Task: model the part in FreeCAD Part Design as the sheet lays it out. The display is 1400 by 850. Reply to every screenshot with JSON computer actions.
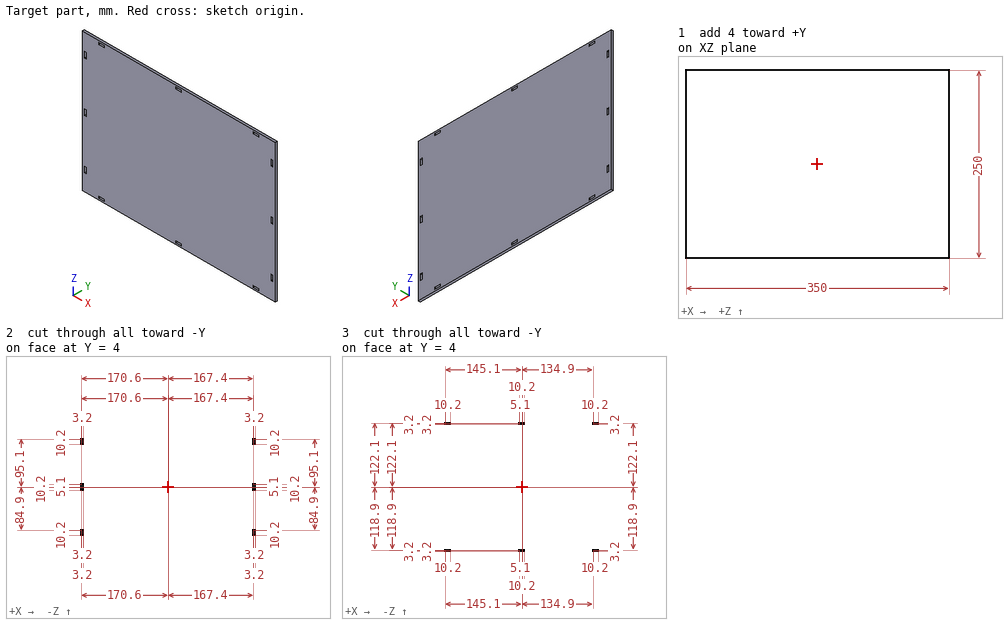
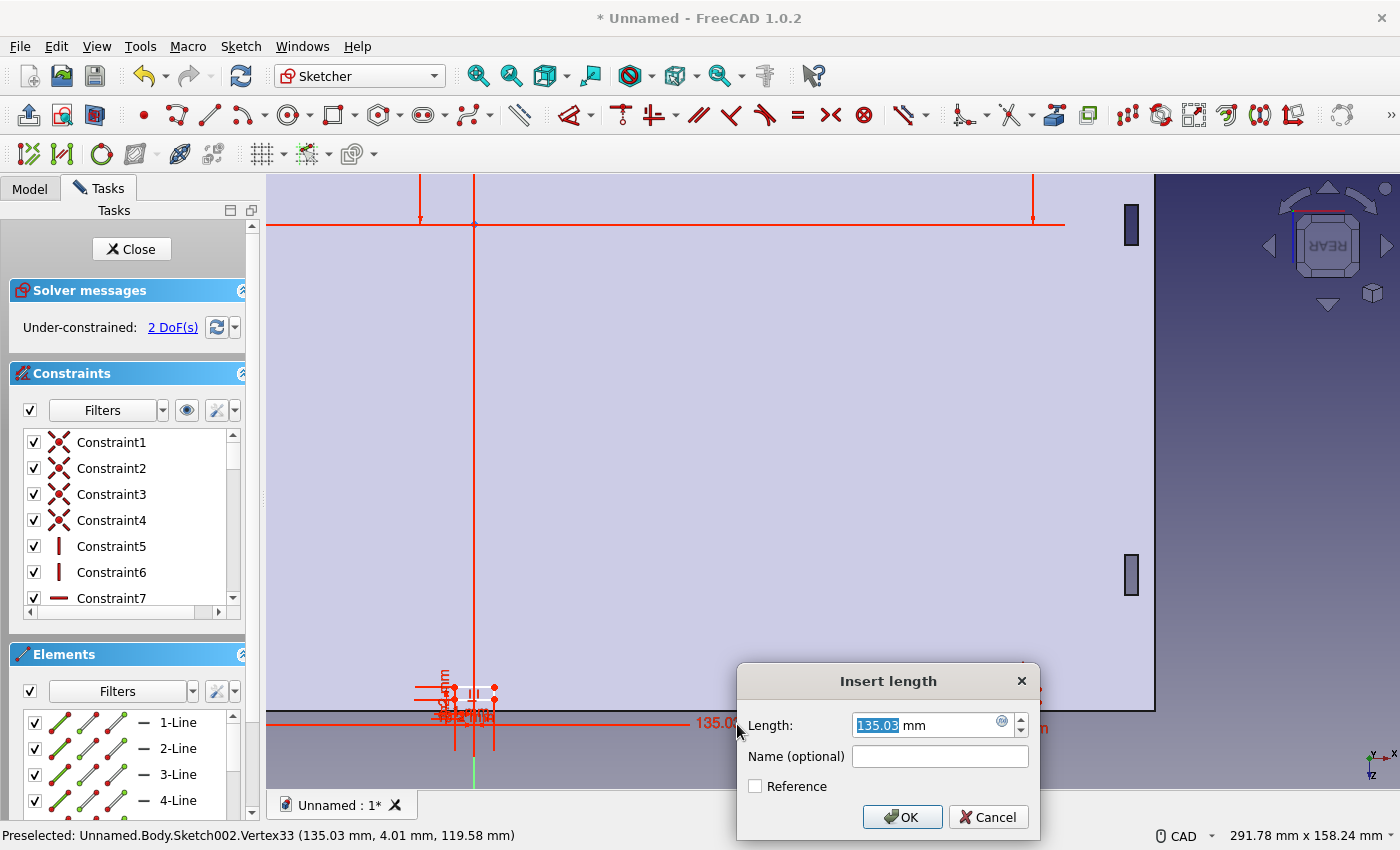
{"action": "type", "text": "134.9"}
{"action": "key", "text": "Return"}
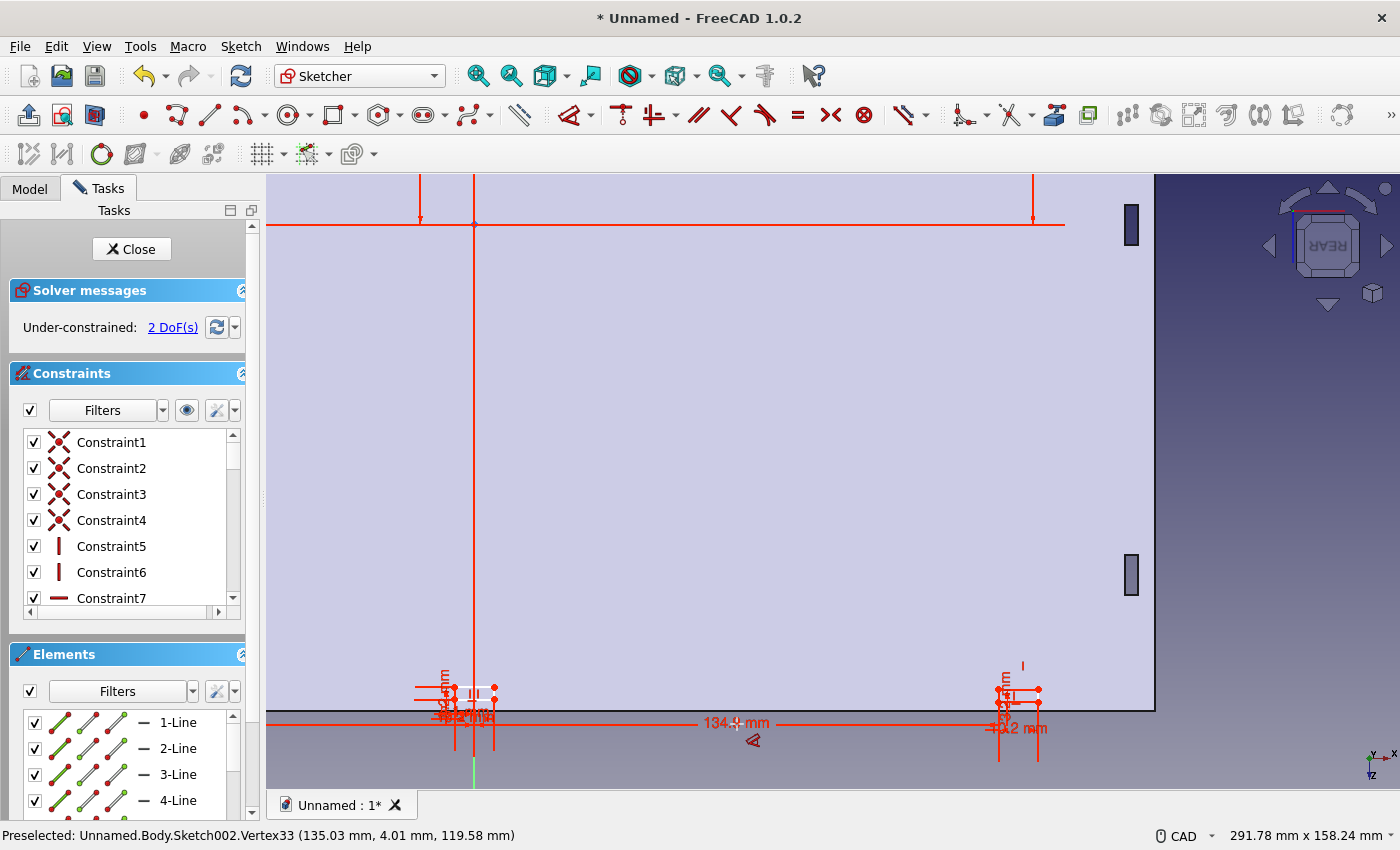
{"action": "left_click", "coordinate": [999, 690]}
{"action": "left_click", "coordinate": [1033, 457]}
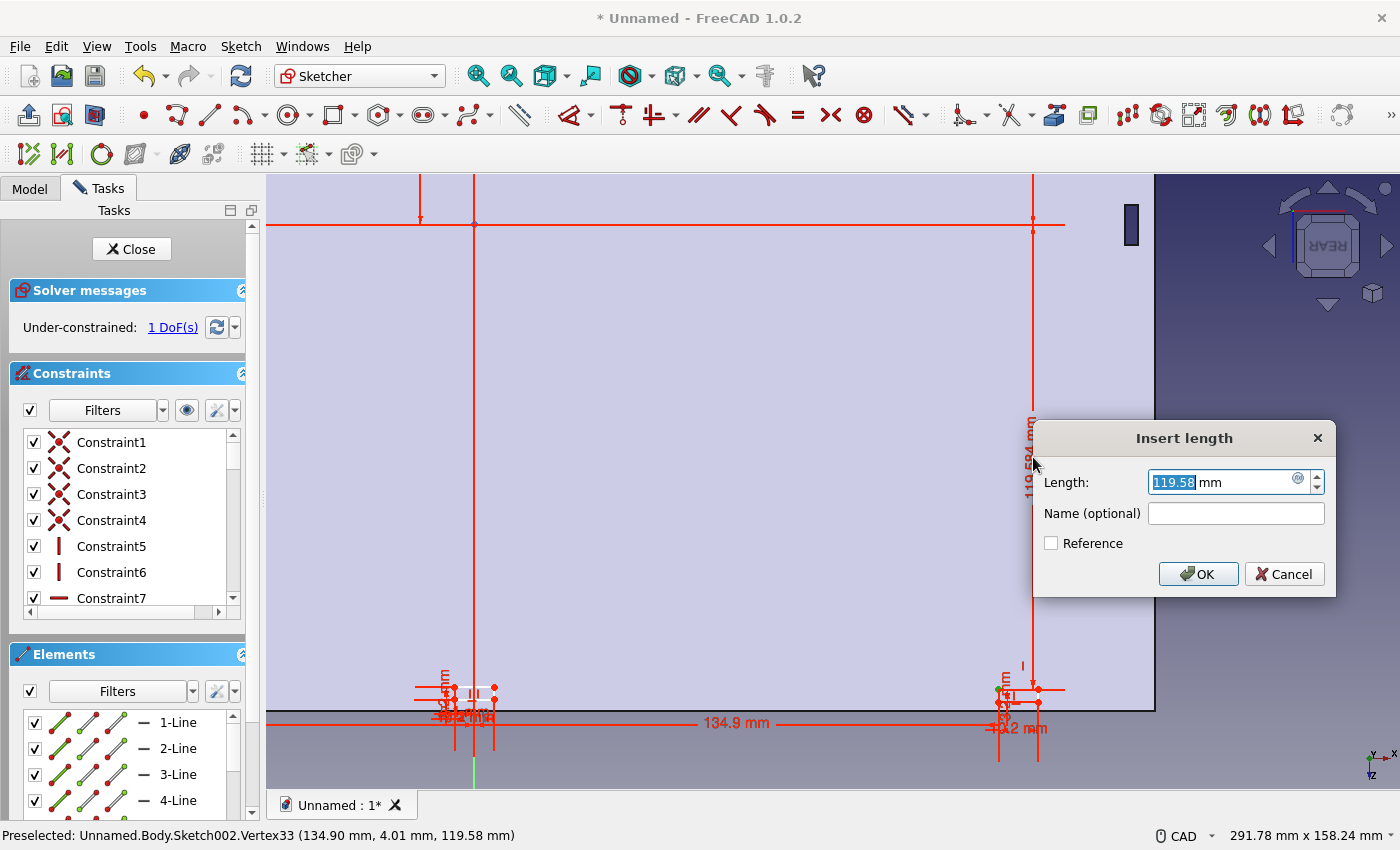
{"action": "type", "text": "118.9"}
{"action": "key", "text": "Return"}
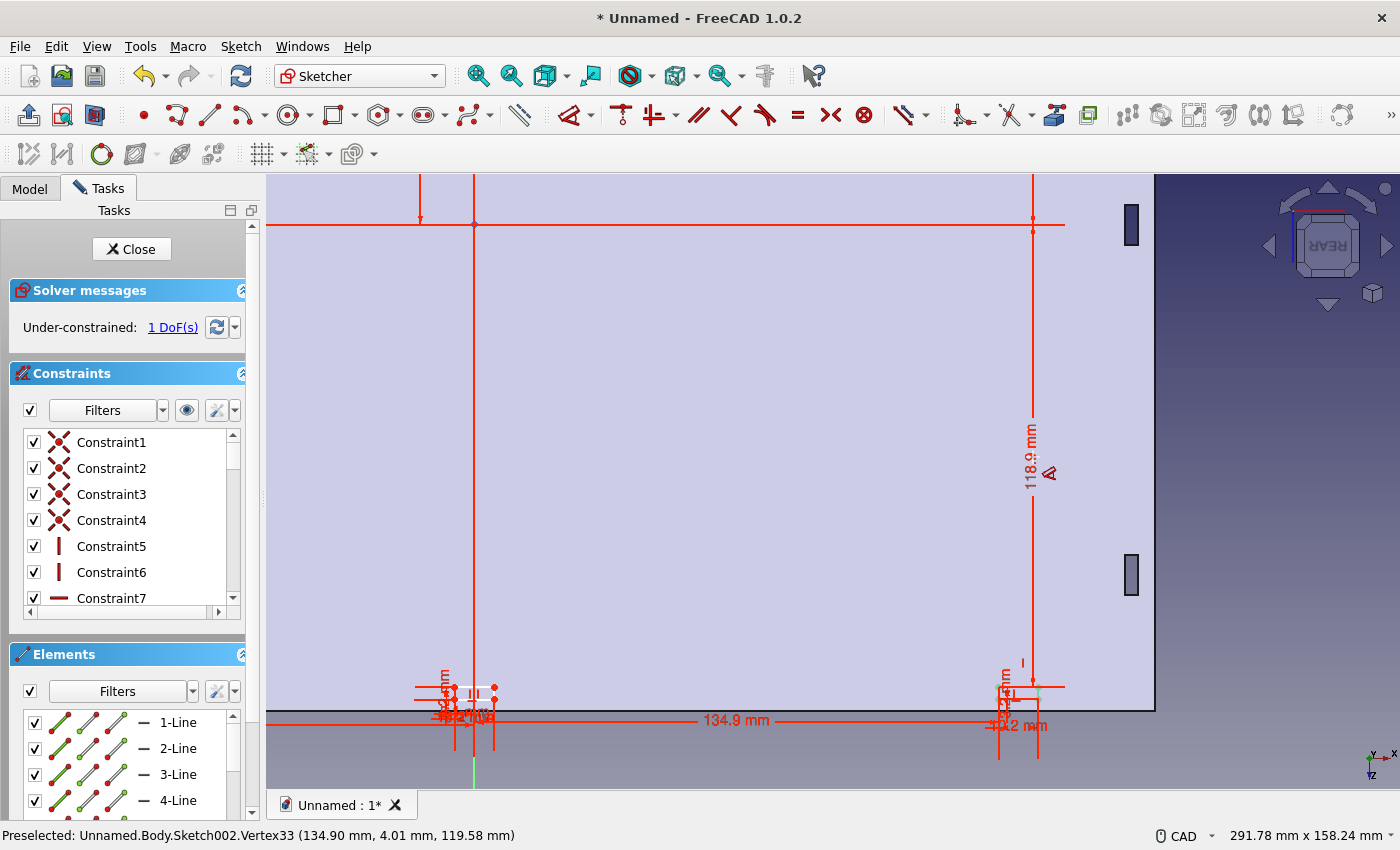
{"action": "left_click", "coordinate": [455, 687]}
{"action": "left_click", "coordinate": [421, 456]}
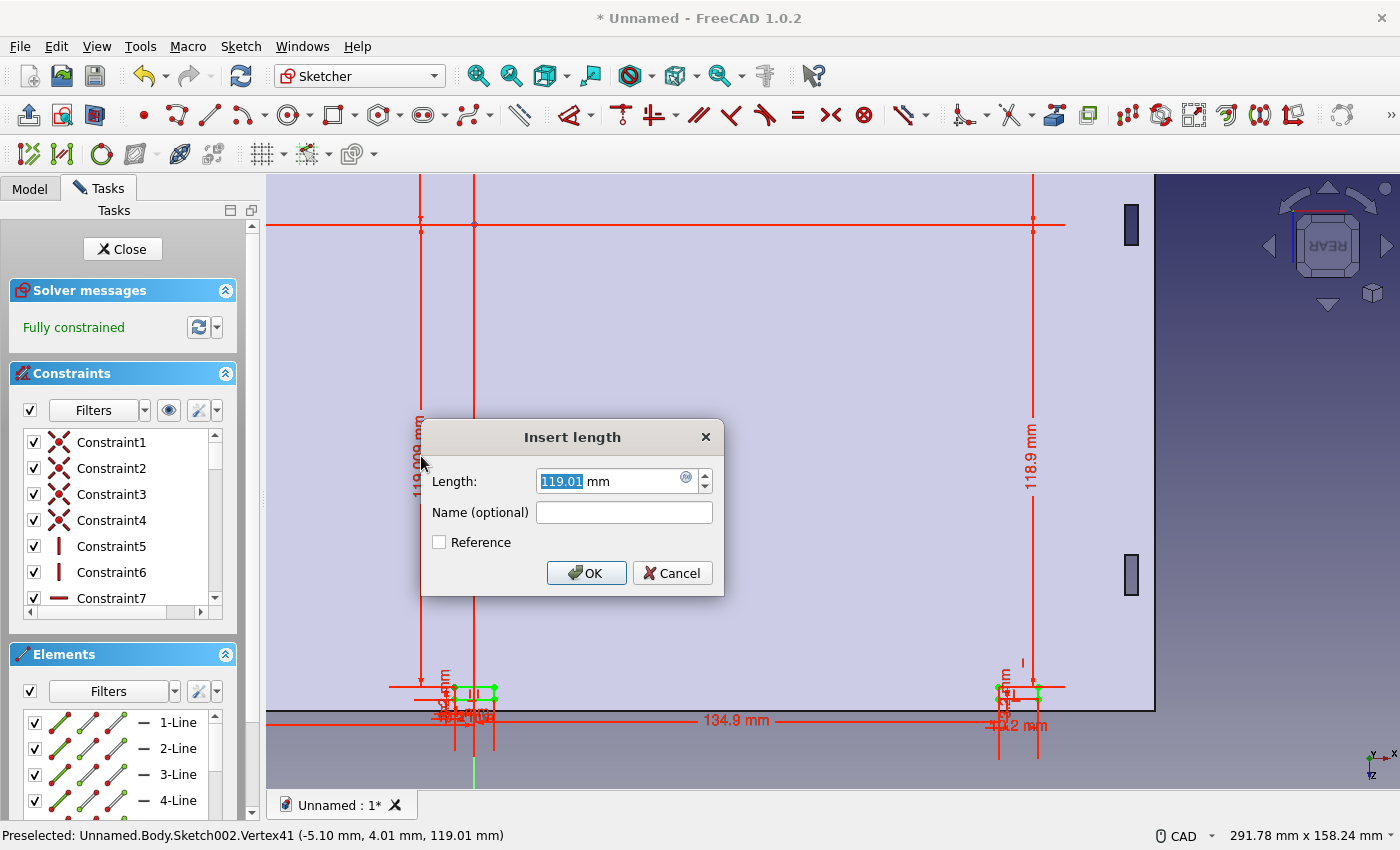
{"action": "type", "text": "118.9"}
{"action": "key", "text": "Return"}
{"action": "key", "text": "Escape"}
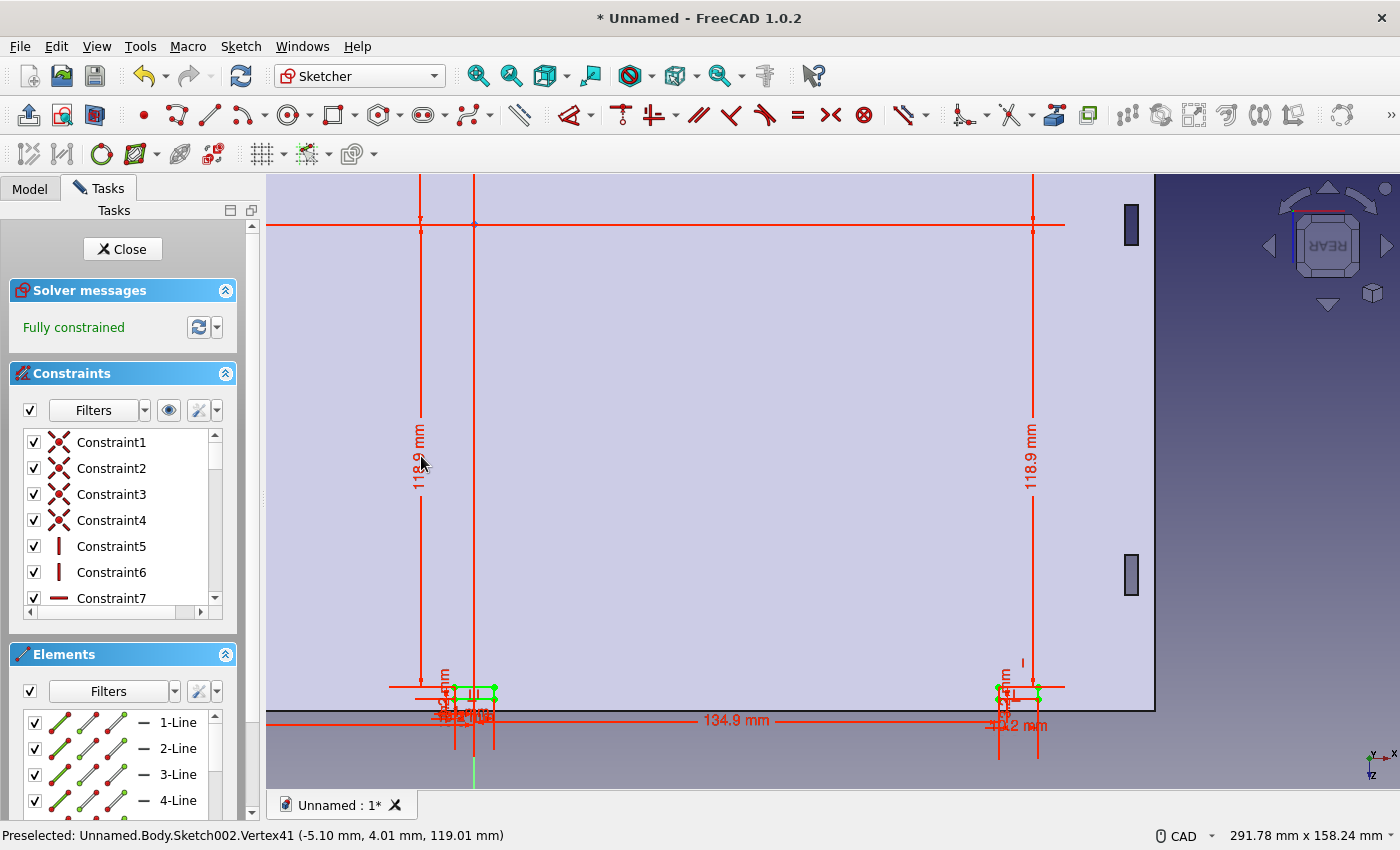
{"action": "left_click", "coordinate": [123, 249]}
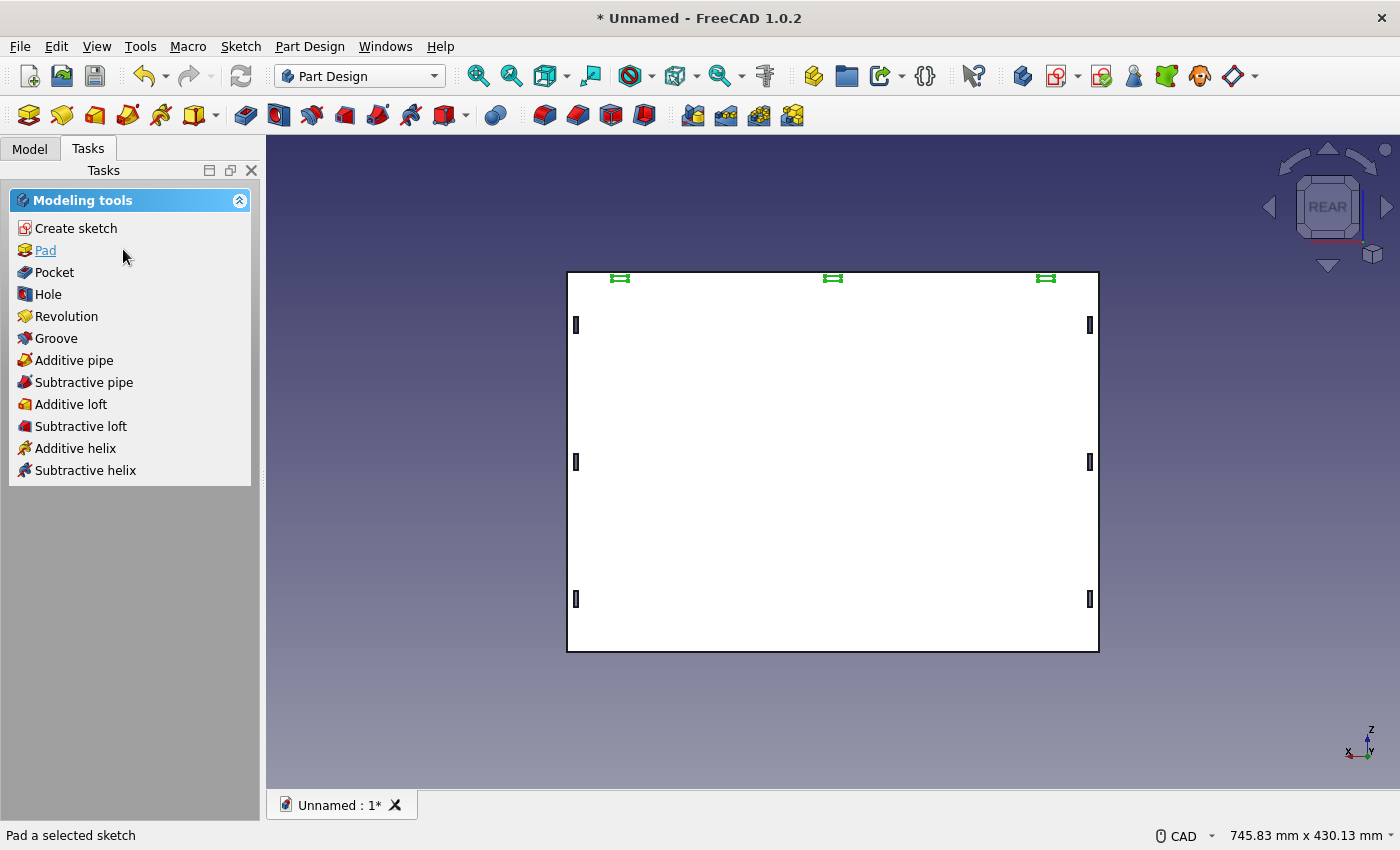
{"action": "left_click", "coordinate": [246, 116]}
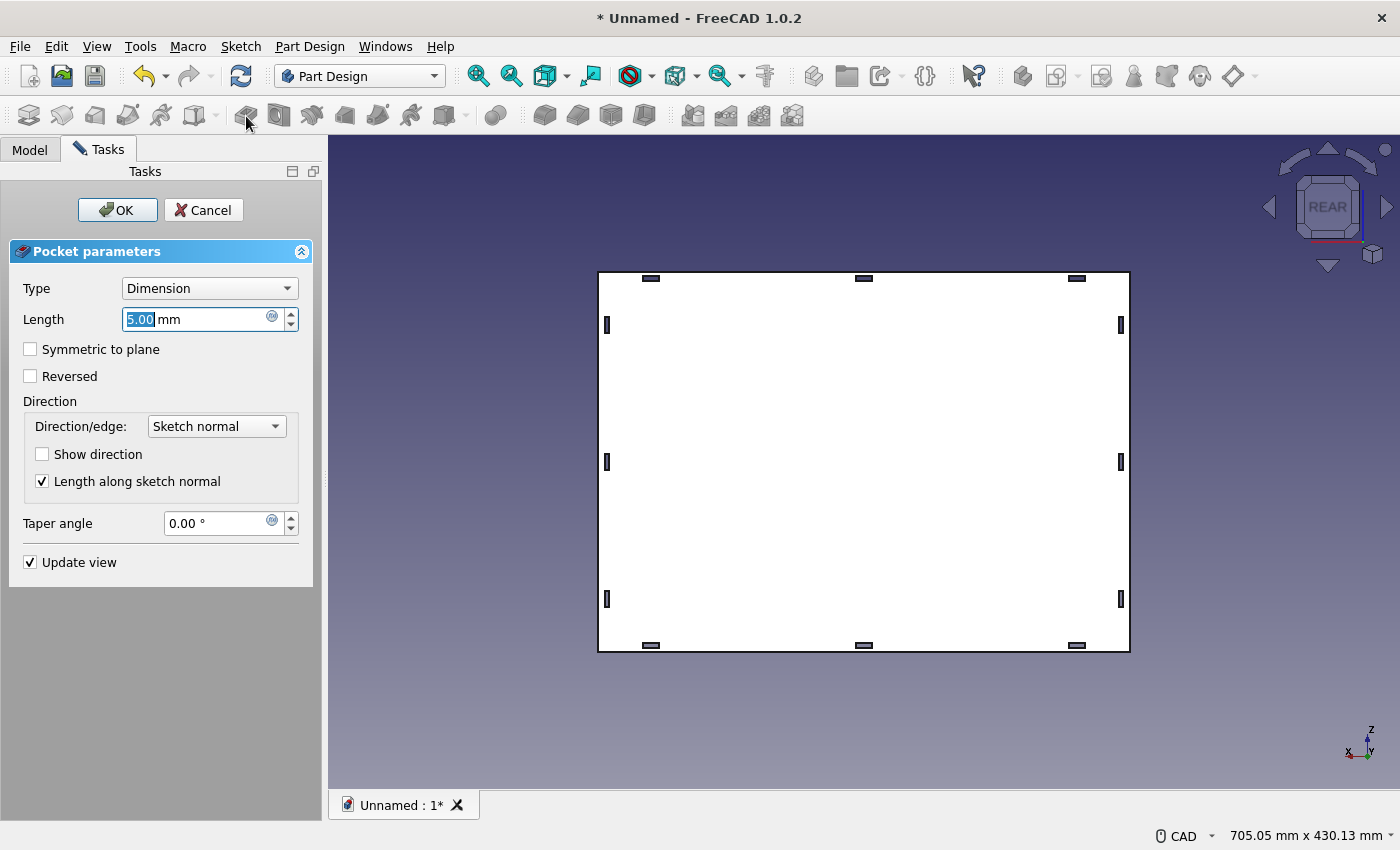
{"action": "left_click", "coordinate": [210, 288]}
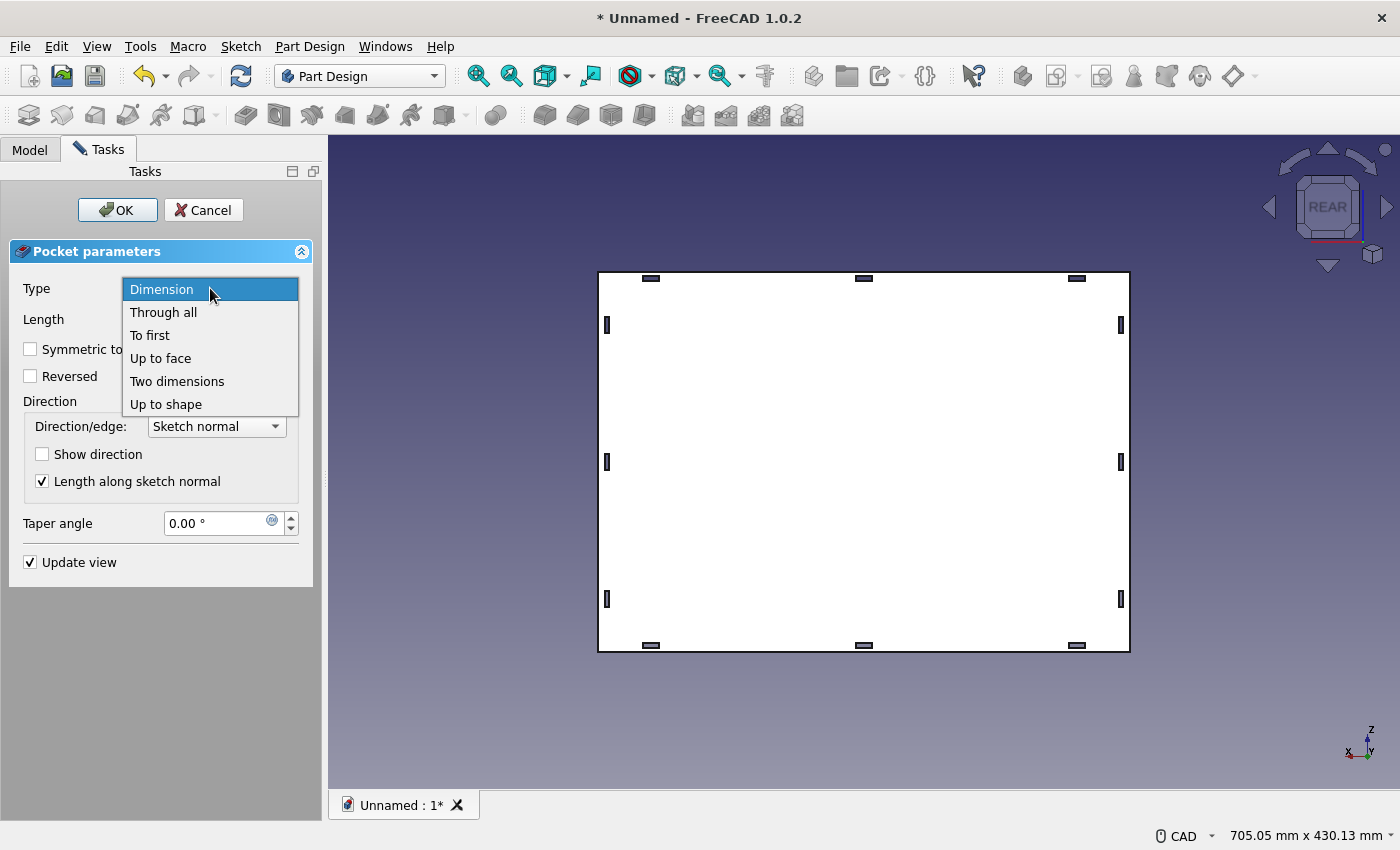
{"action": "left_click", "coordinate": [208, 312]}